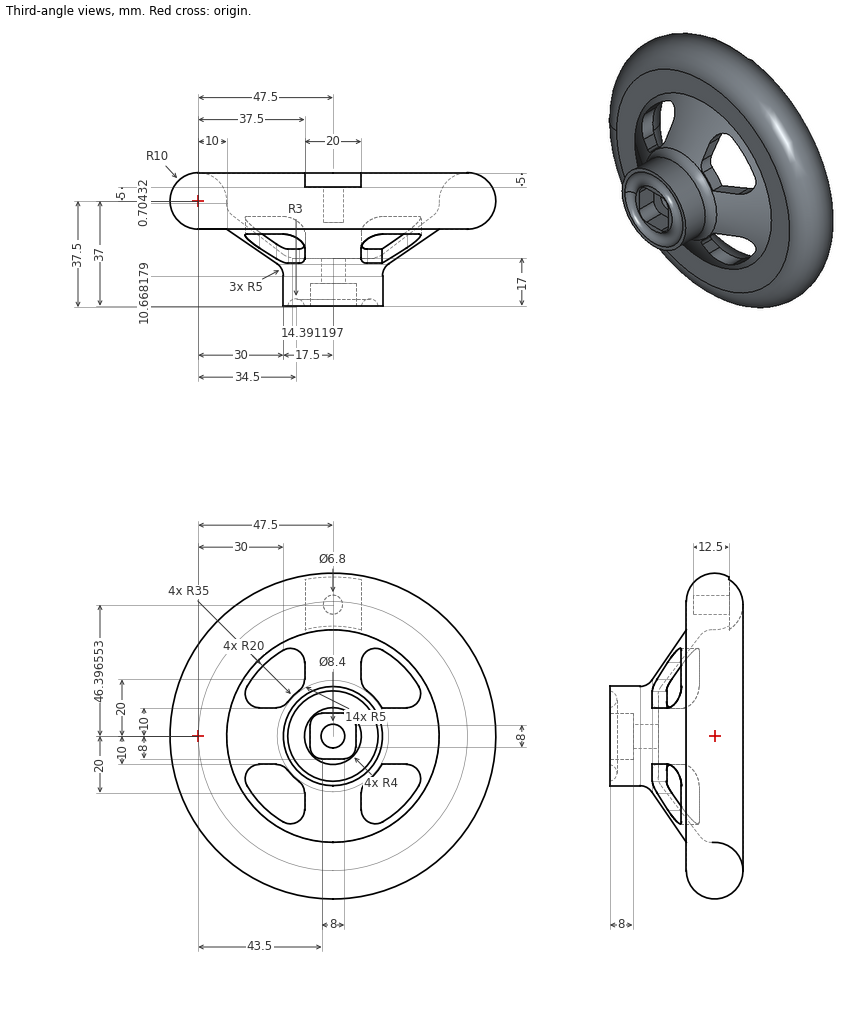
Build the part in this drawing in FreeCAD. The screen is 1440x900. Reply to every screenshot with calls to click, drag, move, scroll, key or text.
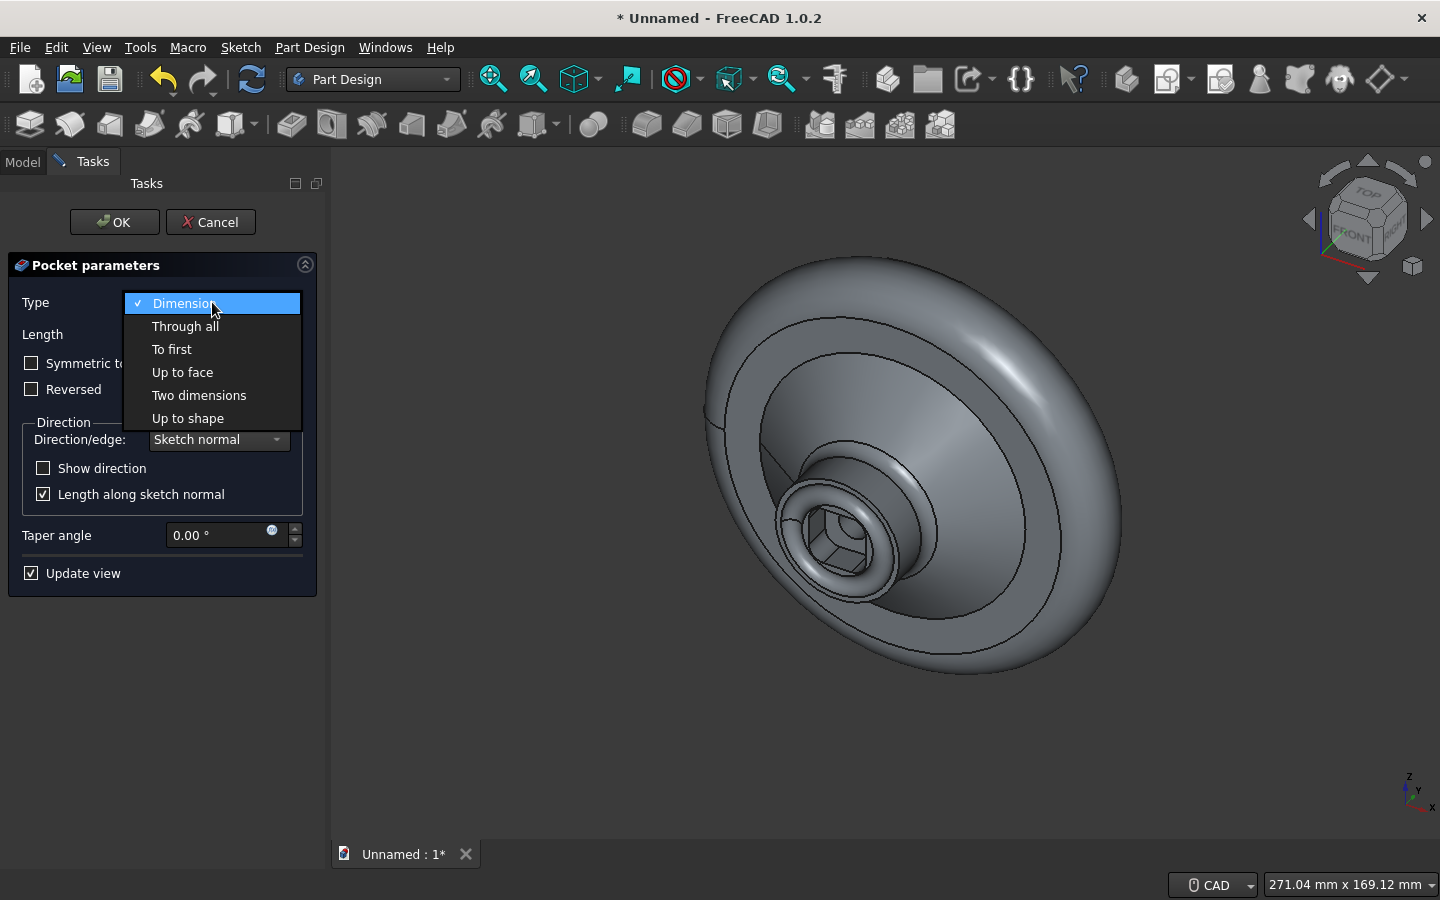
click(212, 326)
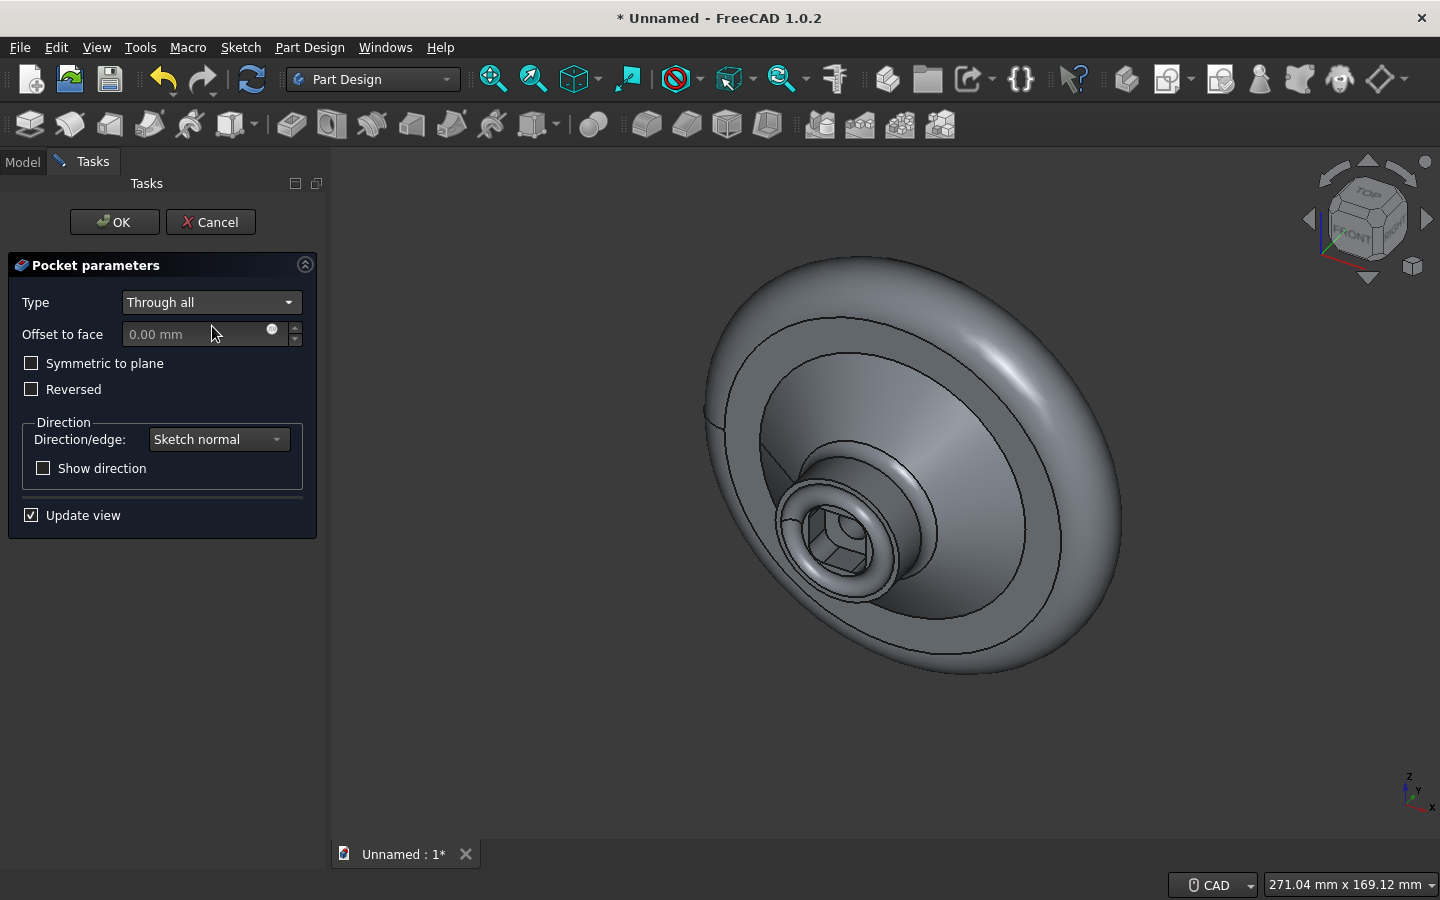
click(30, 389)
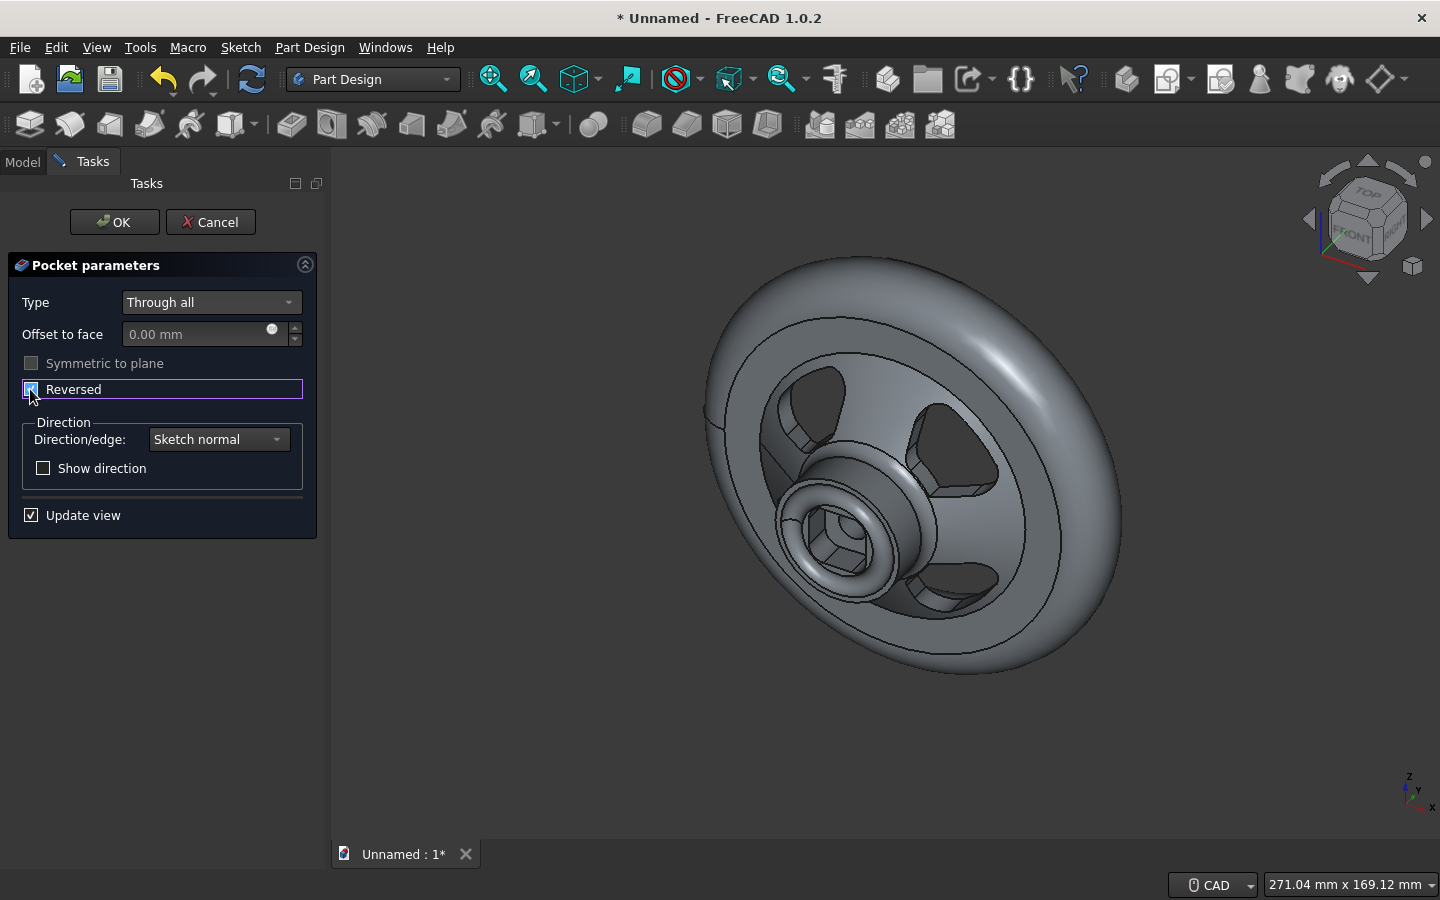
click(115, 222)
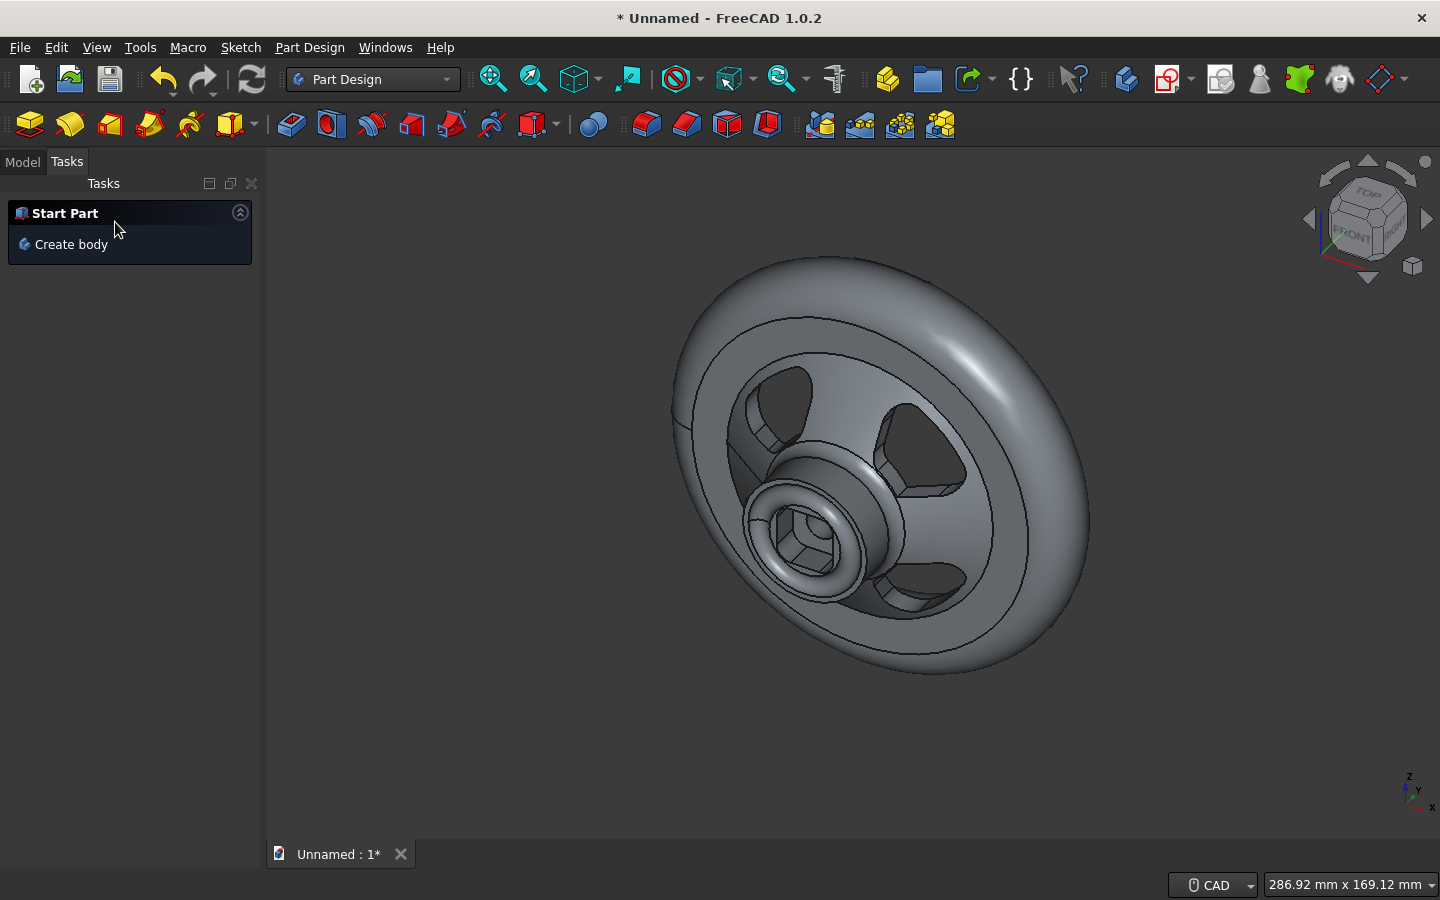
key(4)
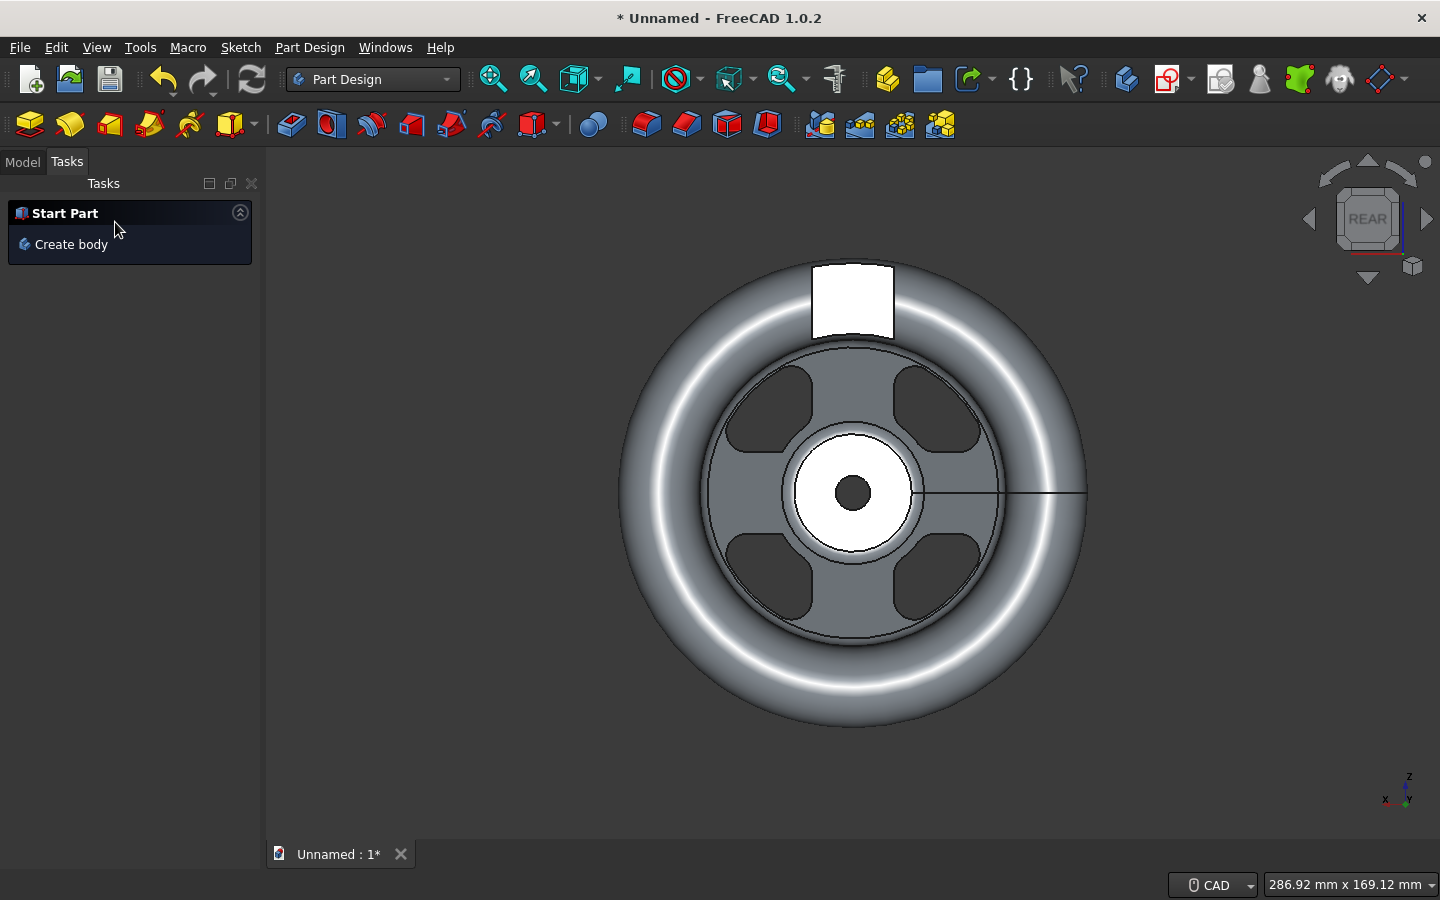
click(853, 300)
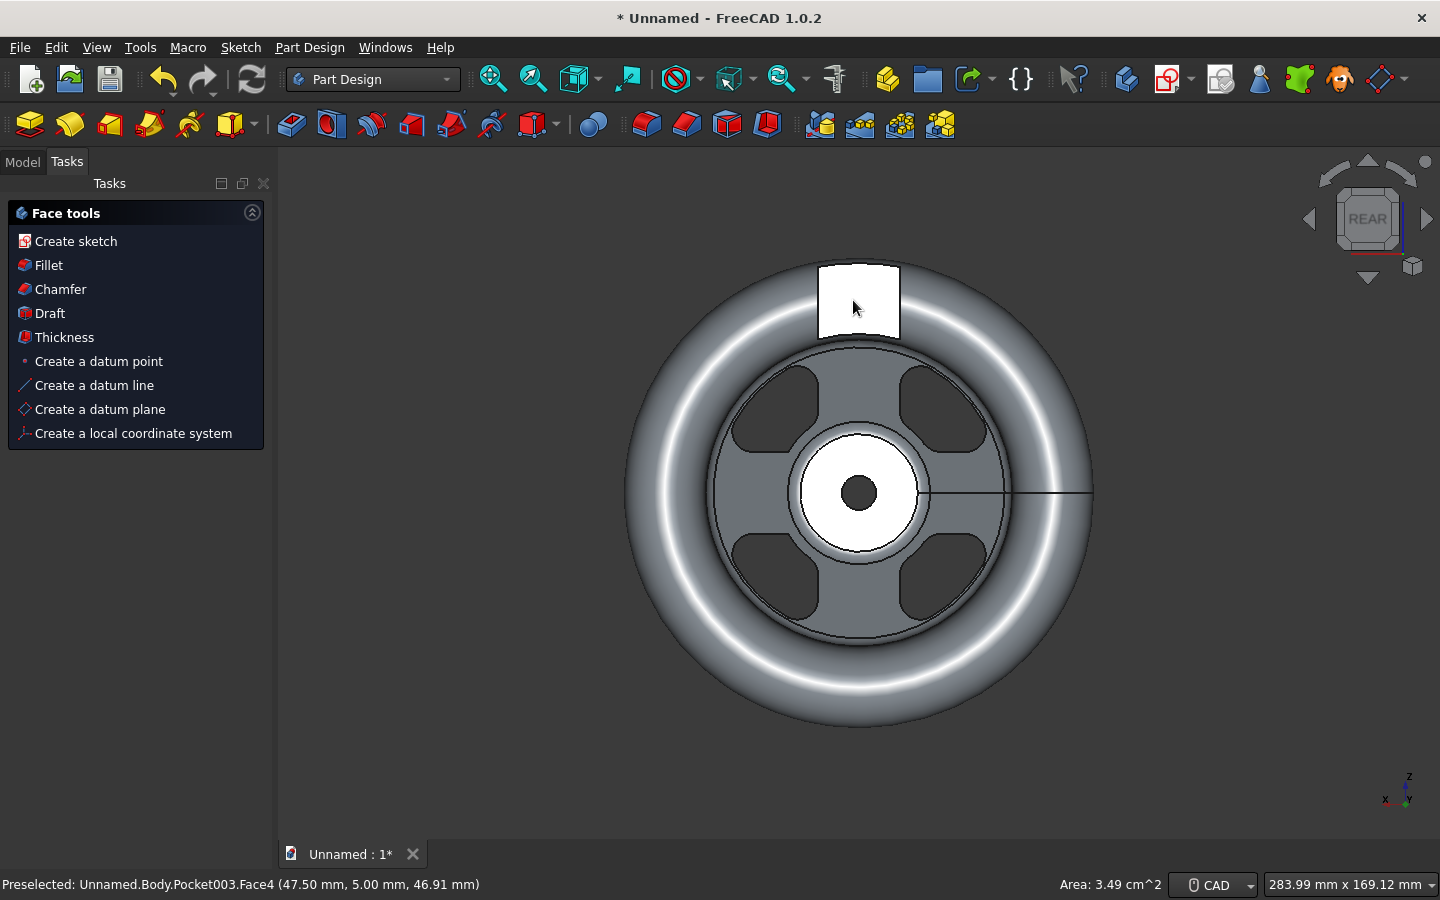
click(1168, 80)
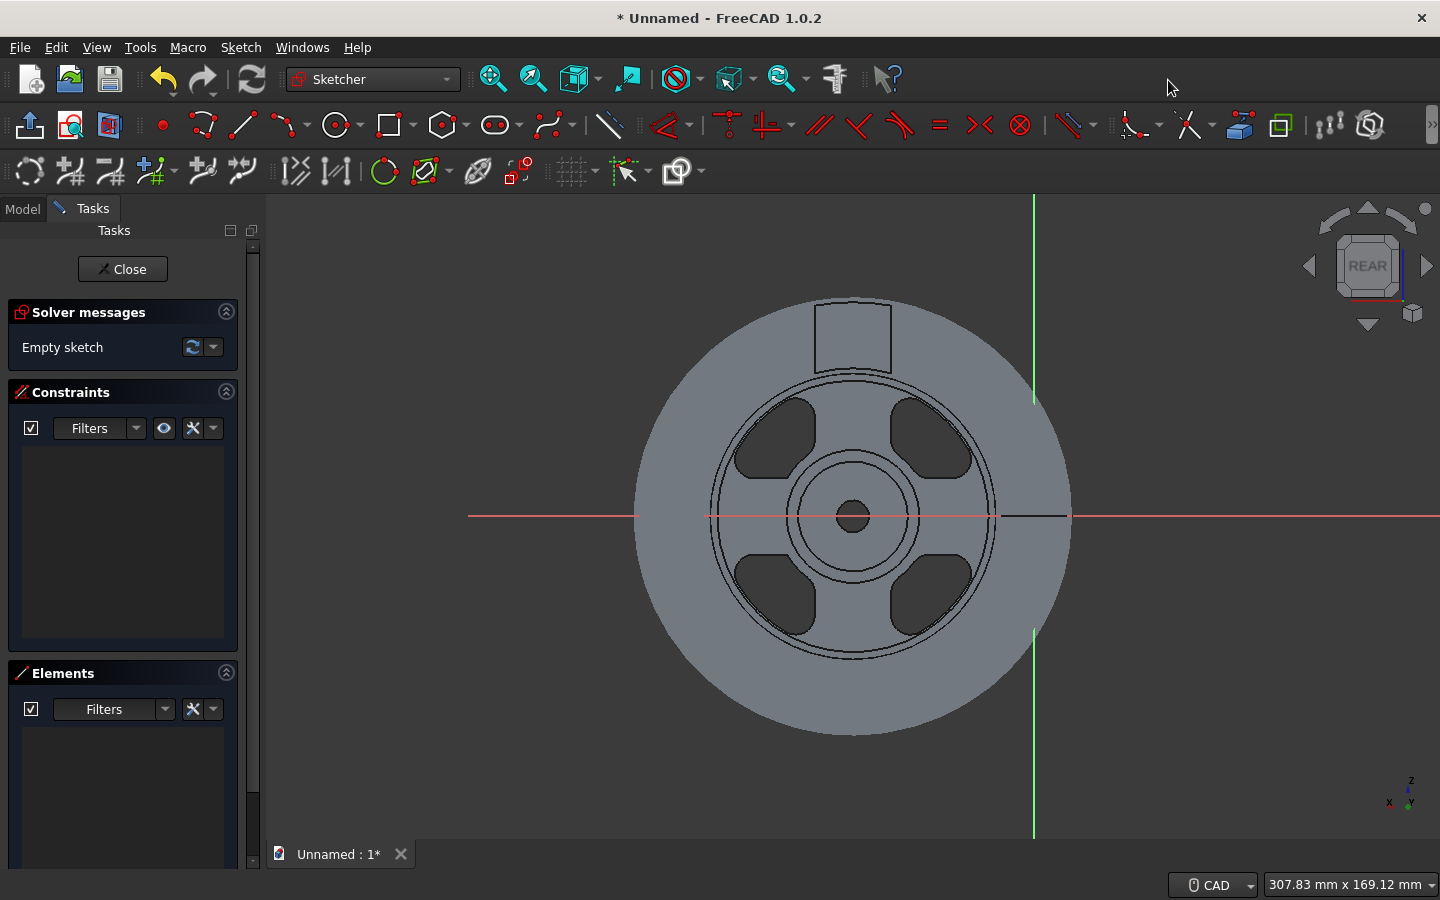
click(110, 126)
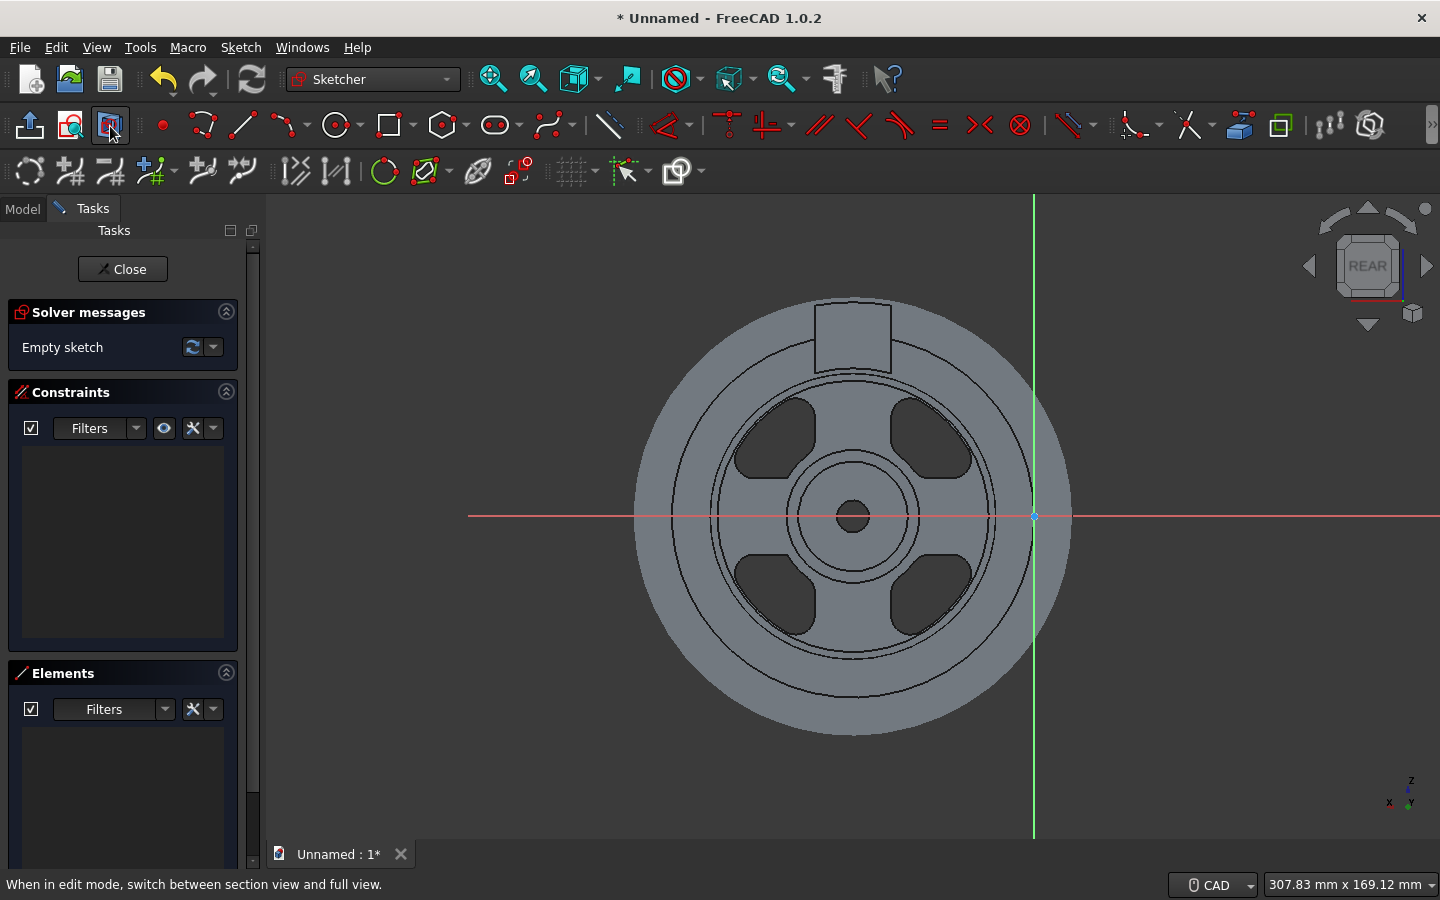
scroll(857, 328, up, 14)